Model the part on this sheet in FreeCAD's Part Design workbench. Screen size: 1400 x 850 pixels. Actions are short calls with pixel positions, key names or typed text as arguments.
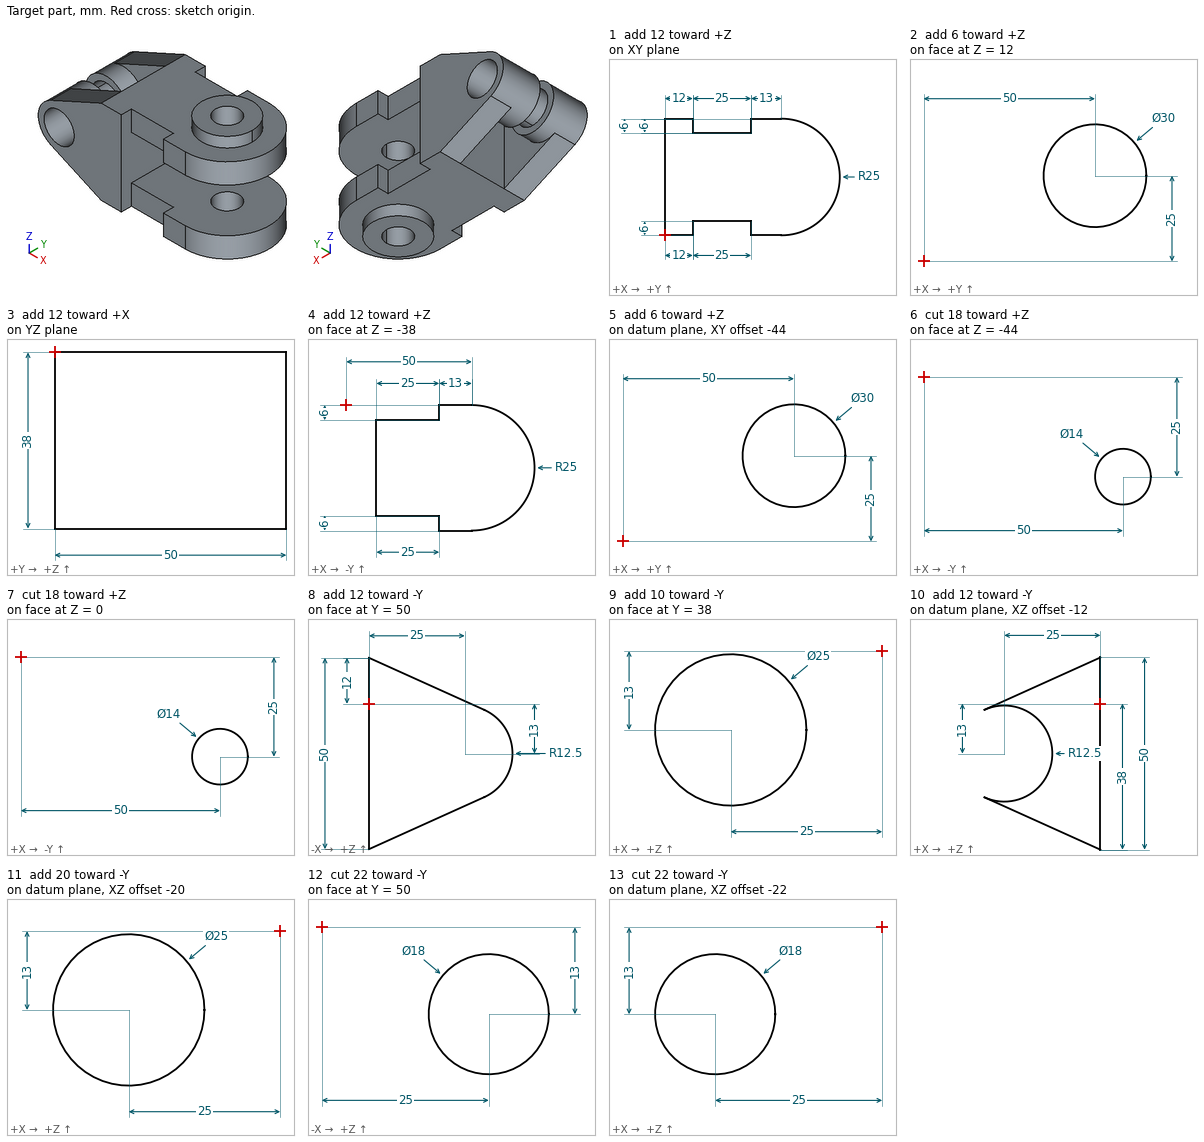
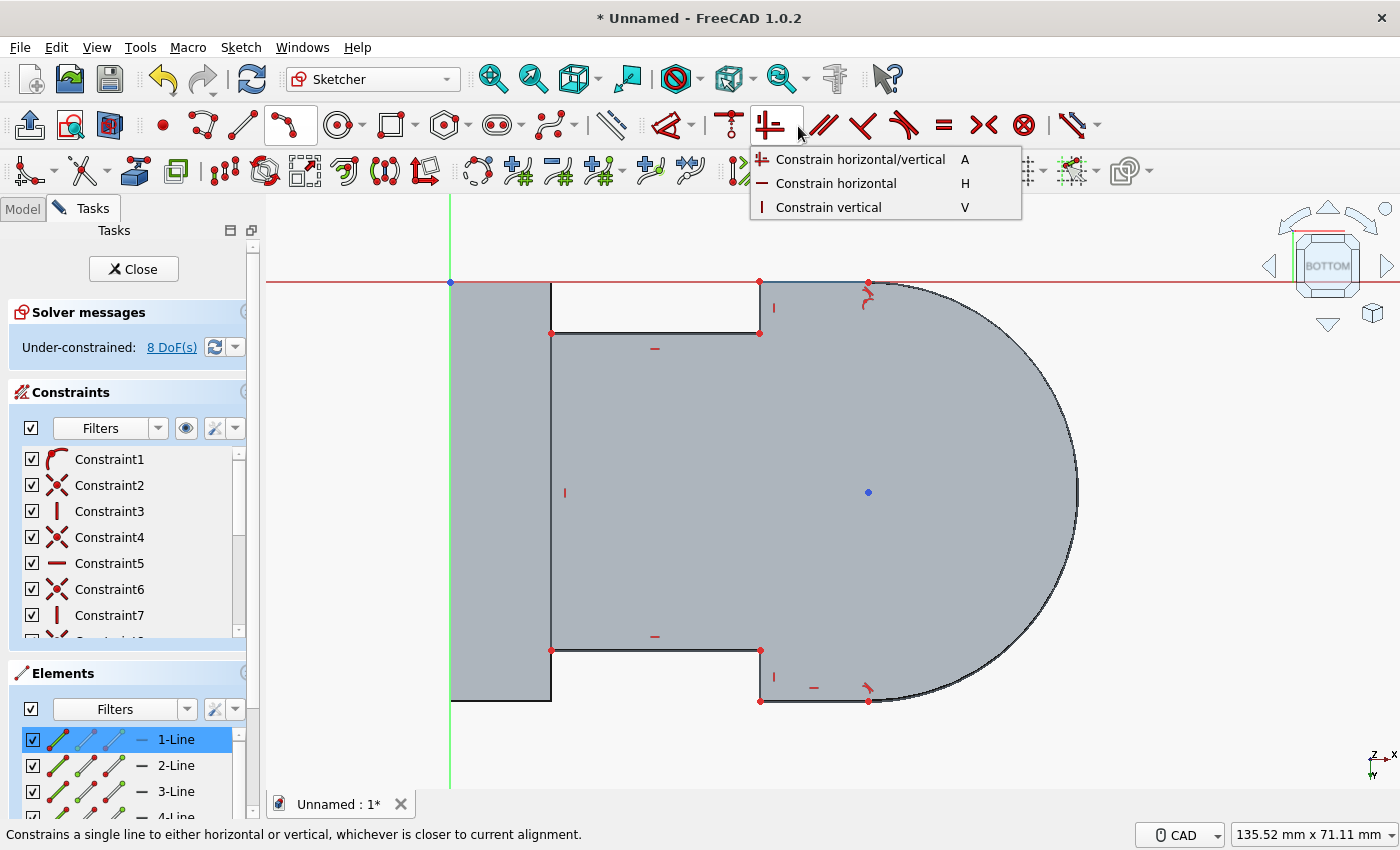
click(886, 183)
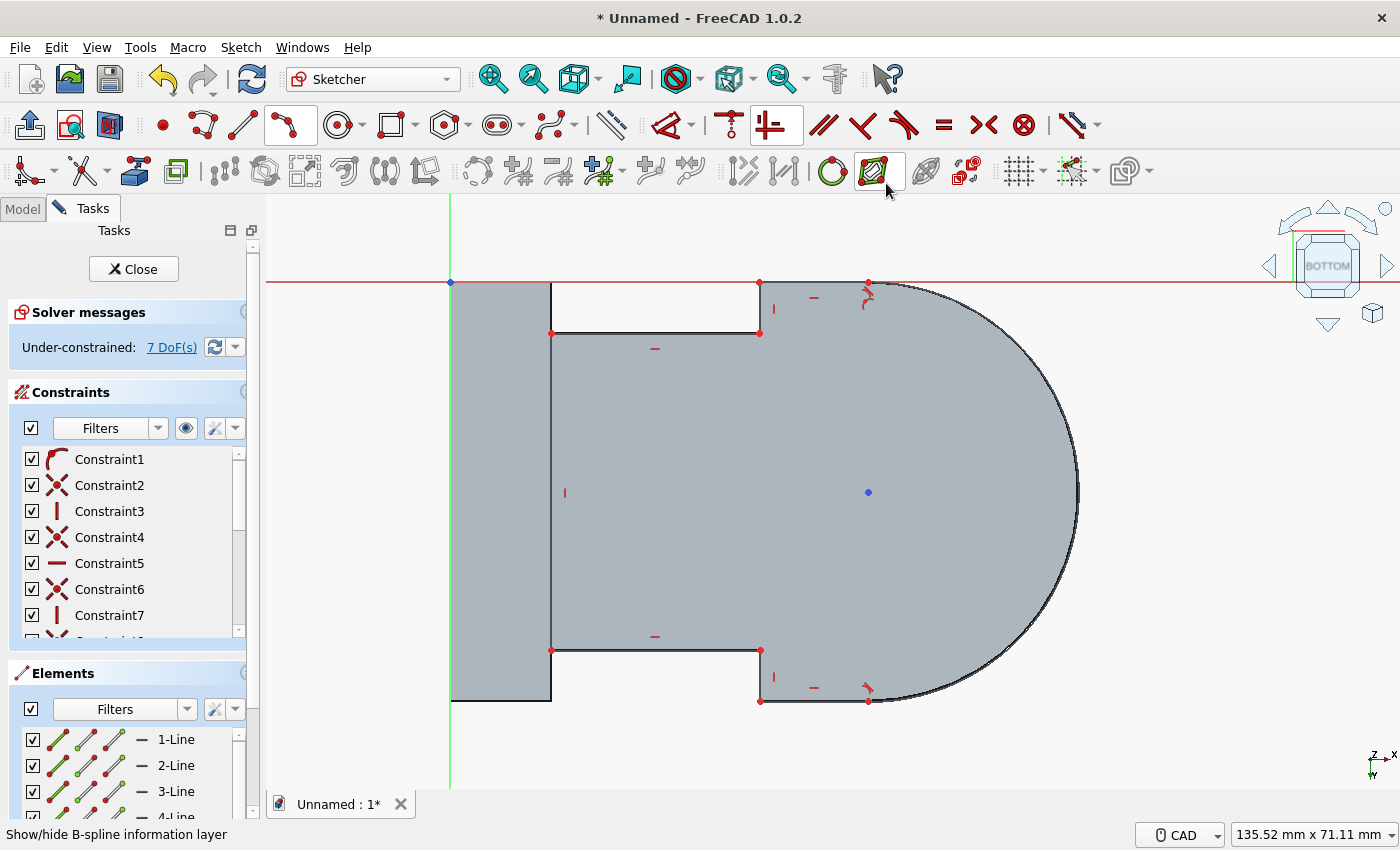
click(666, 126)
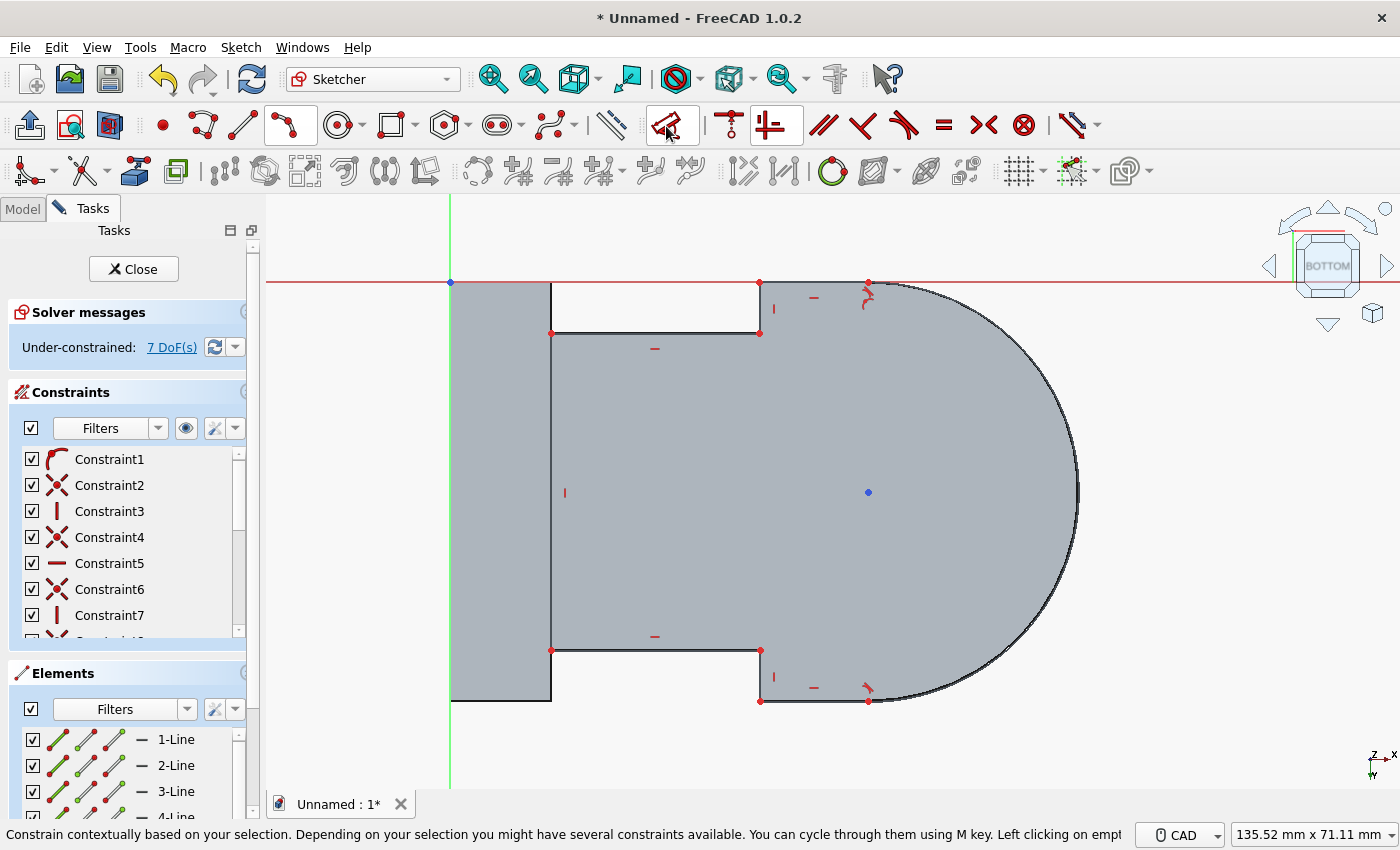
click(1039, 615)
click(1065, 634)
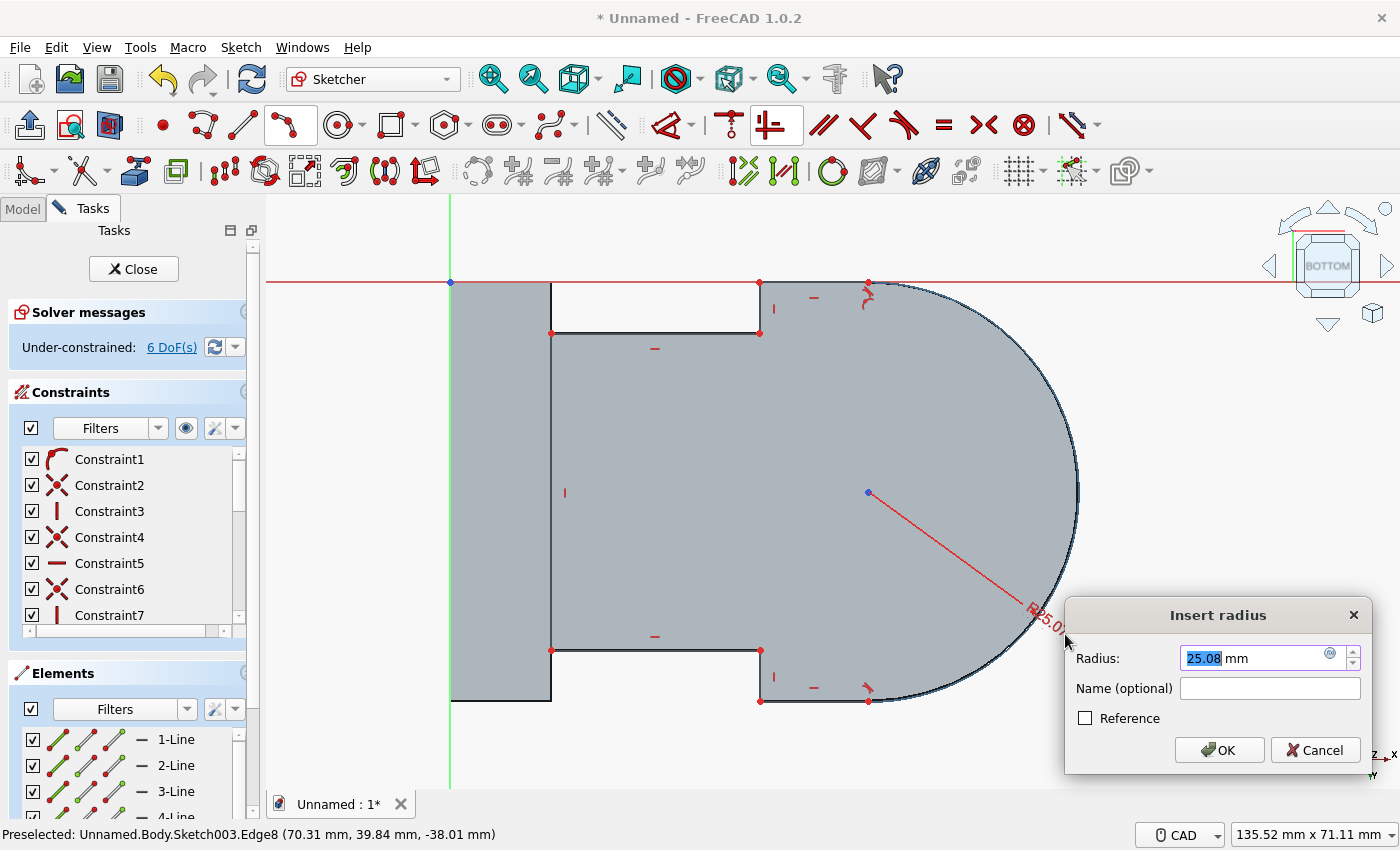
text(25)
key(Return)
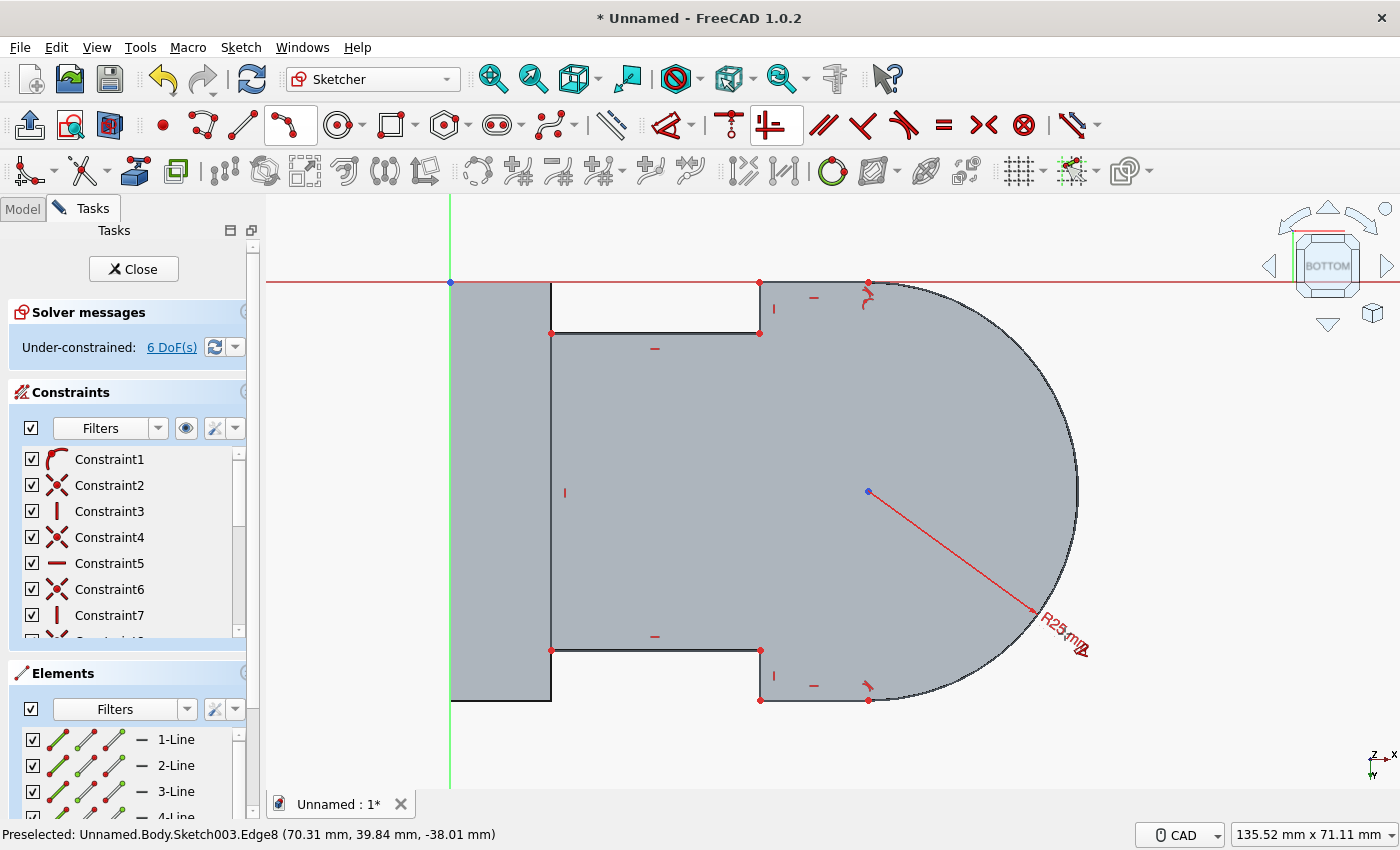
click(760, 298)
click(726, 308)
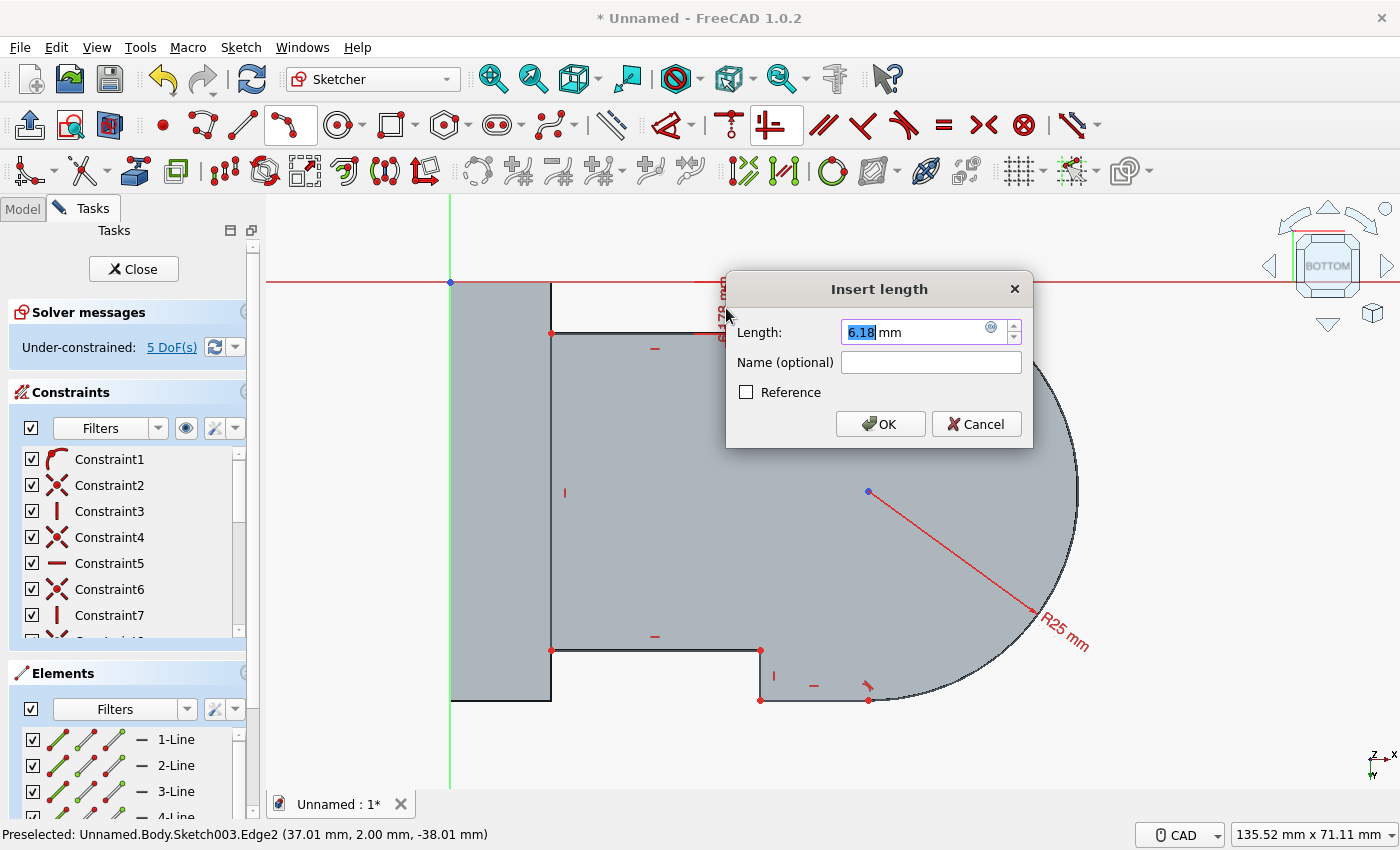
text(6)
key(Return)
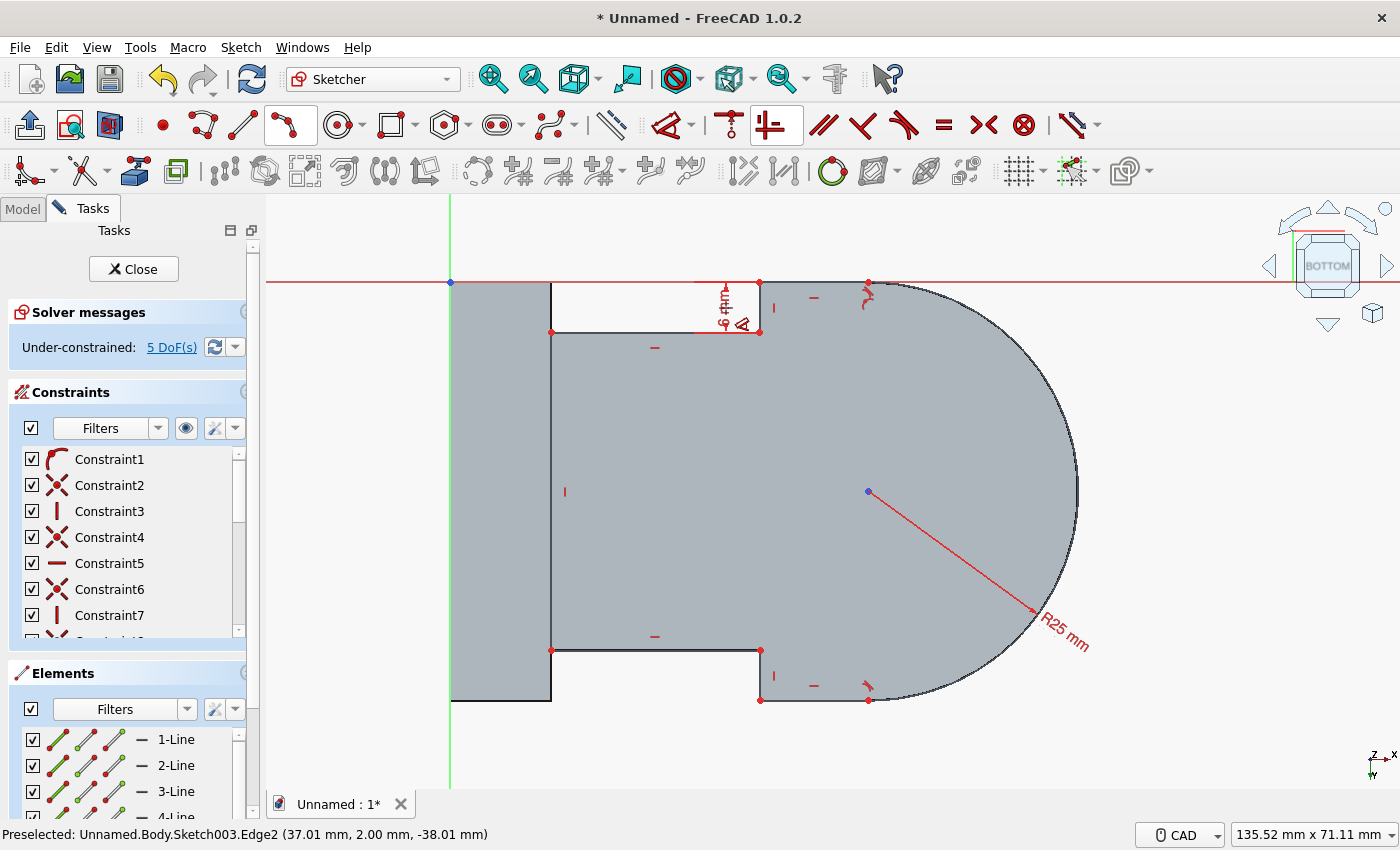
click(760, 666)
click(726, 676)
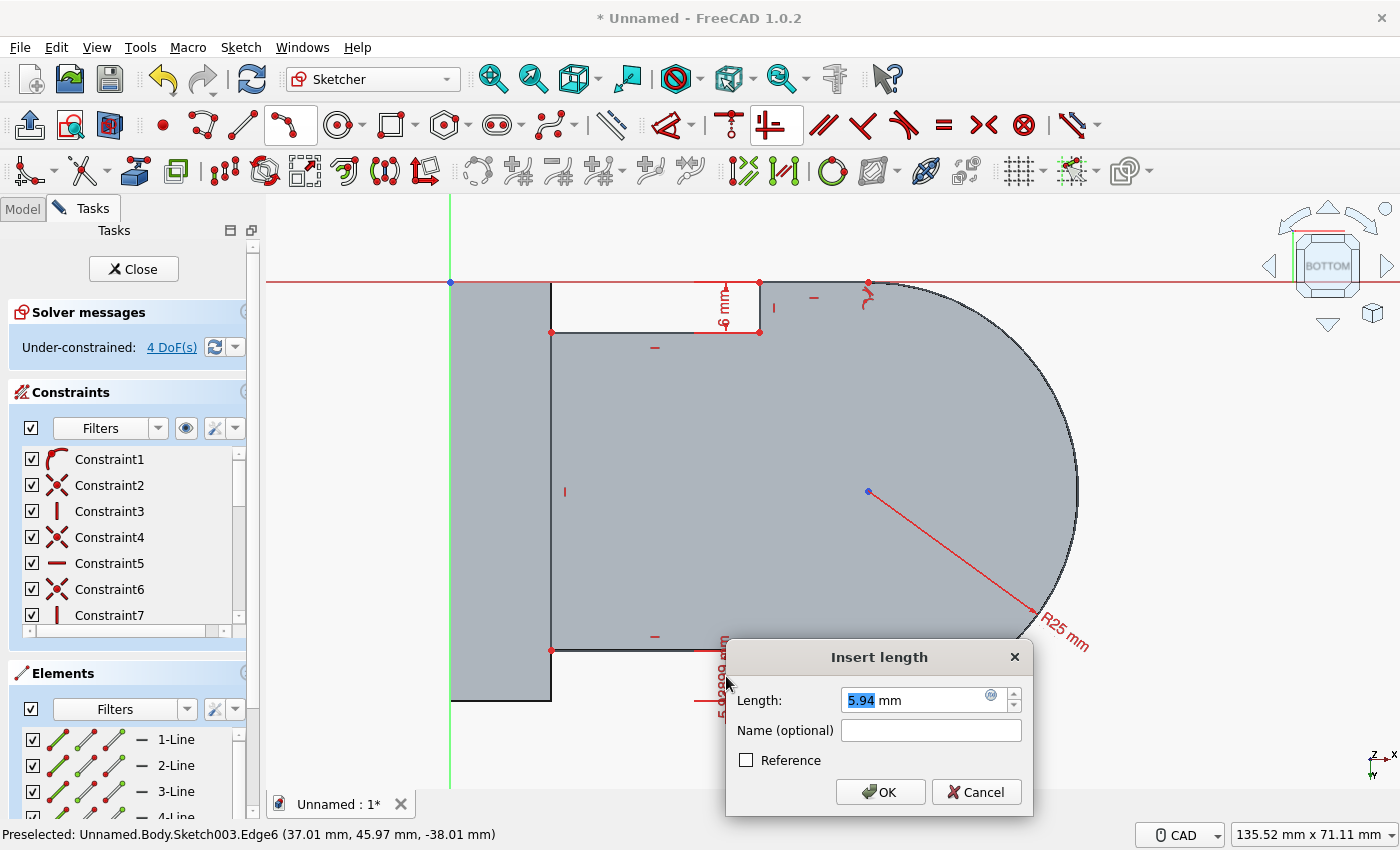
text(6)
key(Return)